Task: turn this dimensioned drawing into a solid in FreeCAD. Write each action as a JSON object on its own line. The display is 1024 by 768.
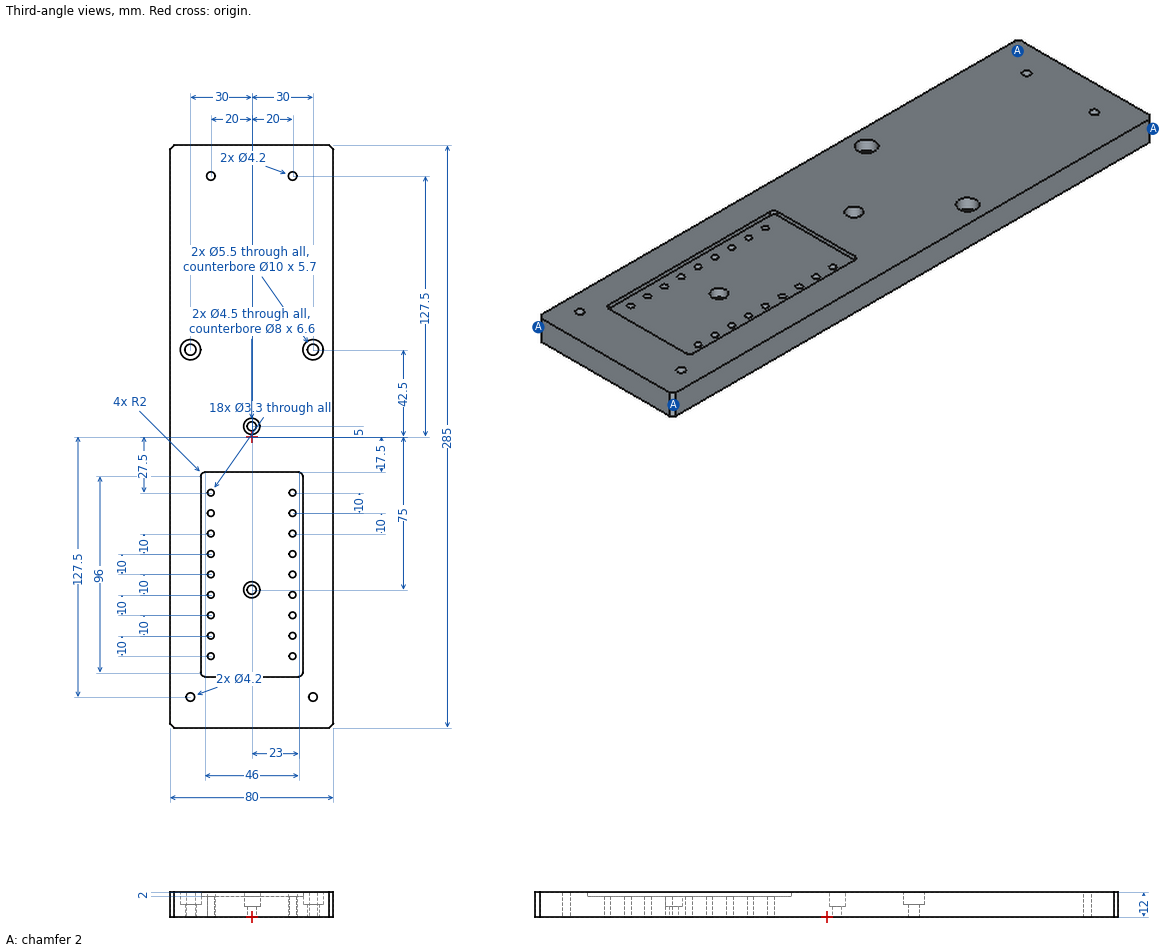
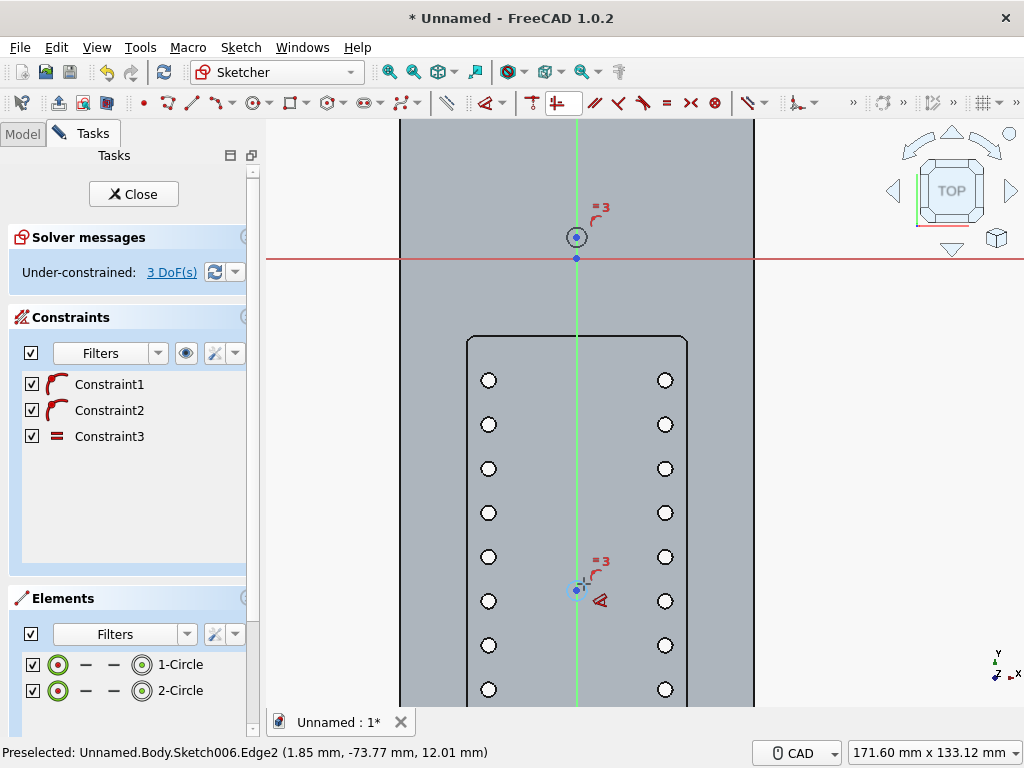
{"action": "scroll", "coordinate": [584, 230], "scroll_direction": "up", "scroll_amount": 4}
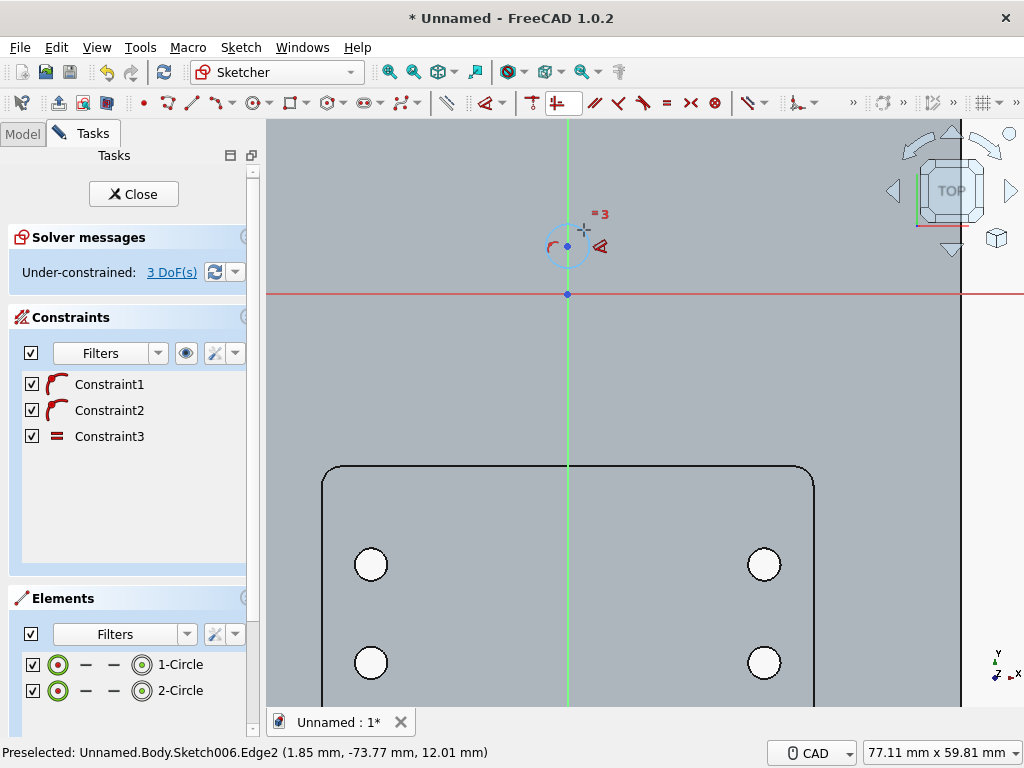
{"action": "left_click", "coordinate": [583, 231]}
{"action": "left_click", "coordinate": [606, 208]}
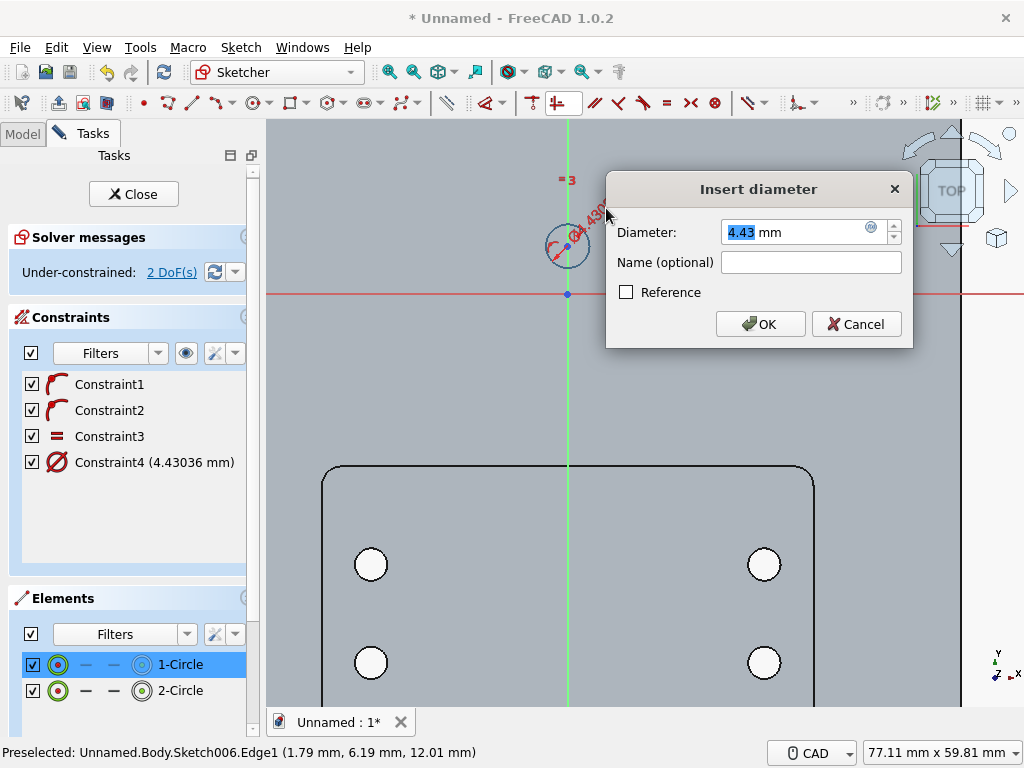
{"action": "type", "text": "4.5"}
{"action": "key", "text": "Return"}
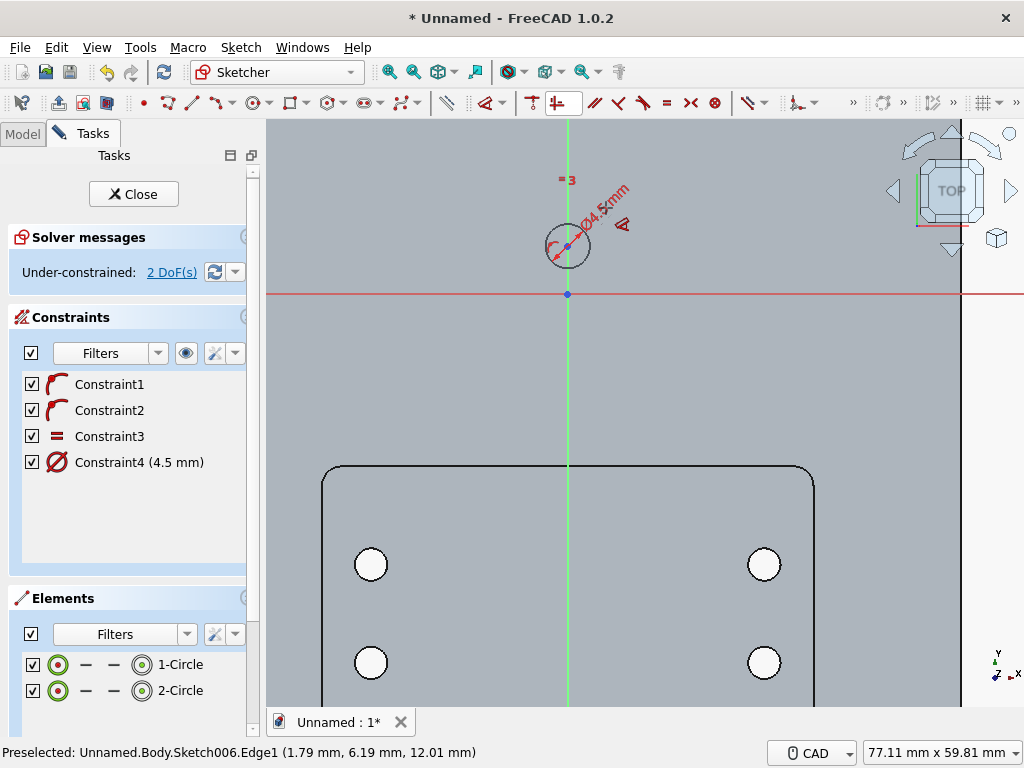
{"action": "left_click", "coordinate": [568, 246]}
{"action": "left_click", "coordinate": [602, 270]}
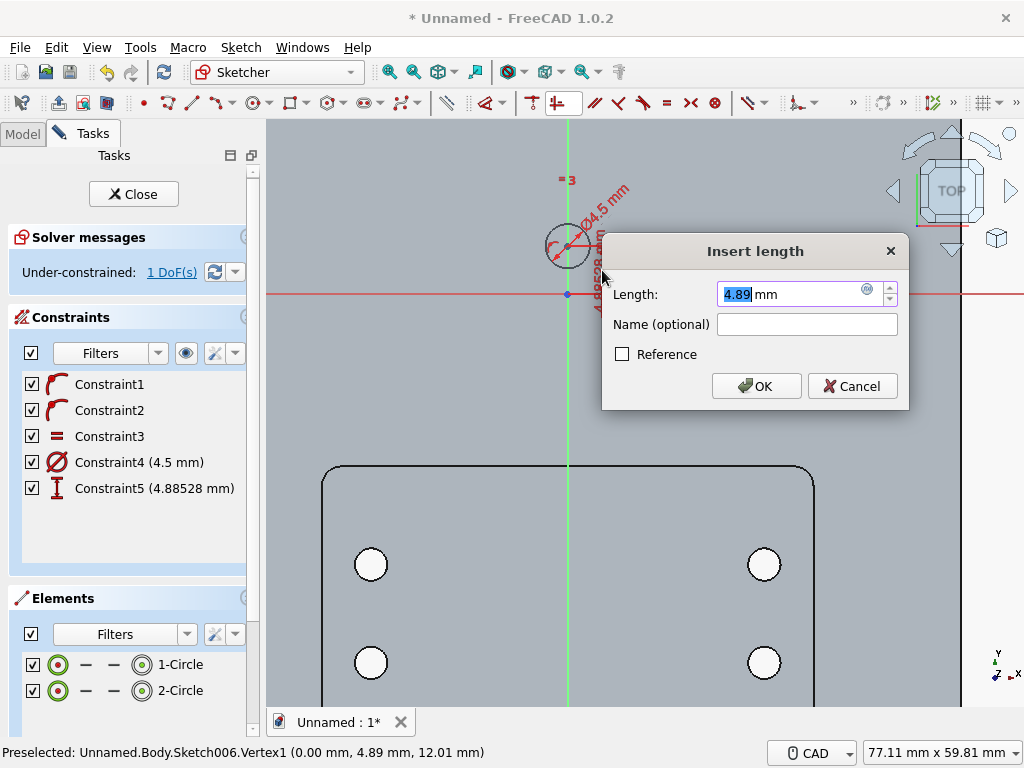
{"action": "type", "text": "5"}
{"action": "key", "text": "Return"}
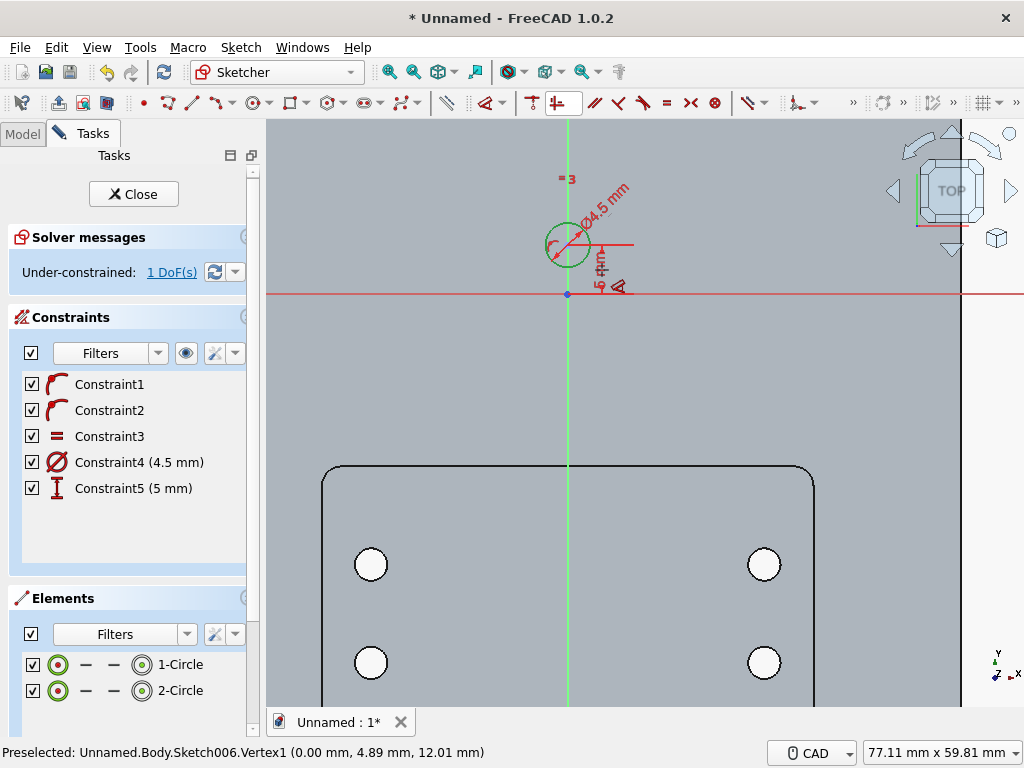
{"action": "scroll", "coordinate": [584, 229], "scroll_direction": "down", "scroll_amount": 4}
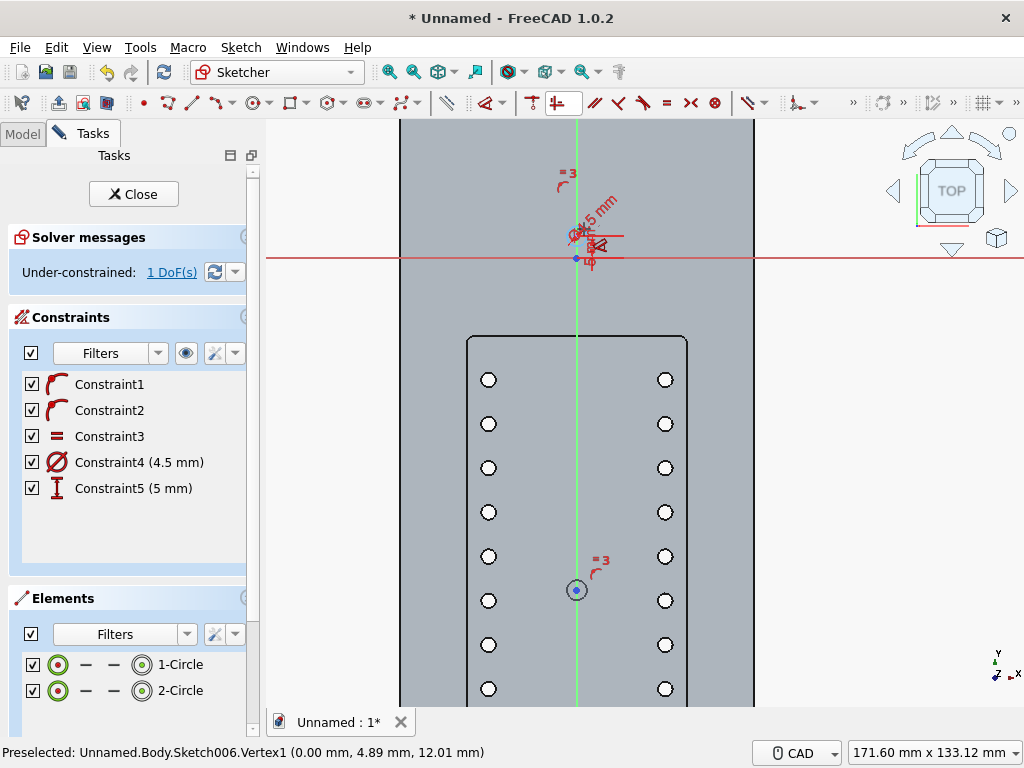
{"action": "left_click", "coordinate": [577, 590]}
{"action": "left_click", "coordinate": [611, 424]}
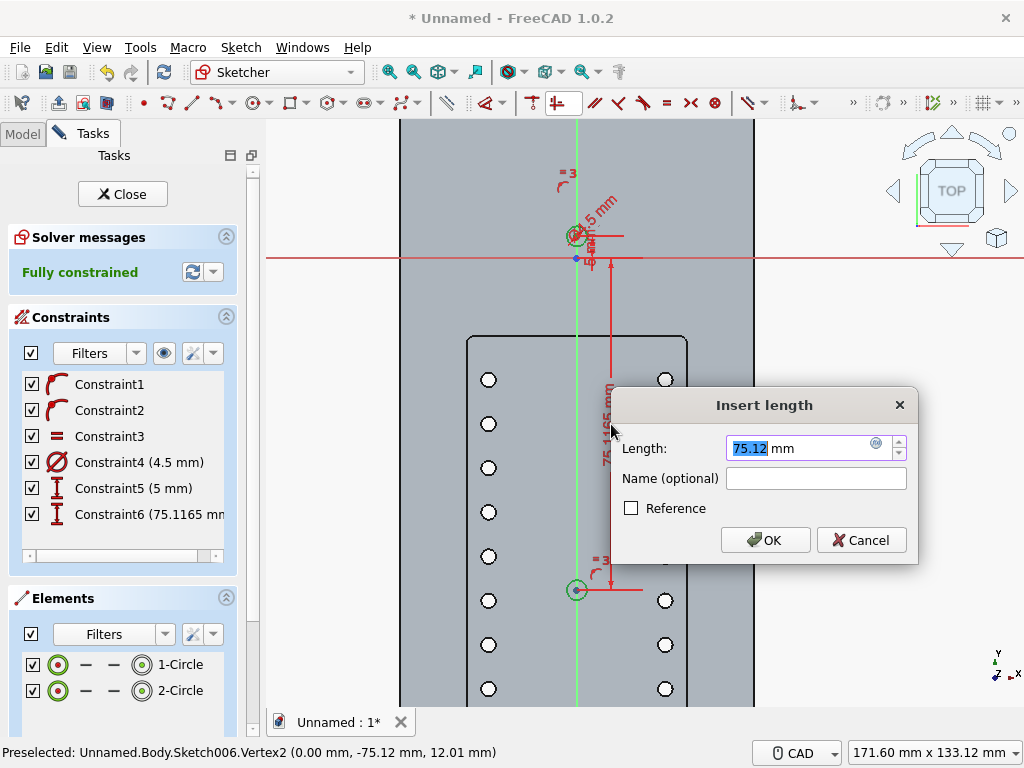
{"action": "type", "text": "75"}
{"action": "key", "text": "Return"}
{"action": "key", "text": "Escape"}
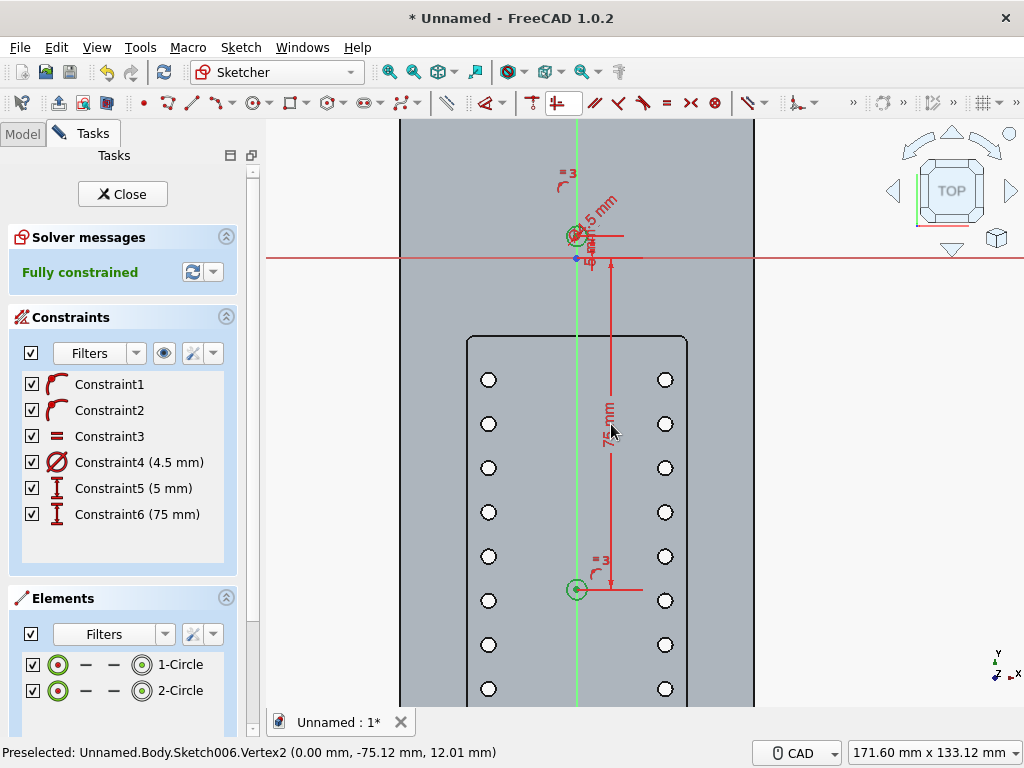
{"action": "left_click", "coordinate": [123, 194]}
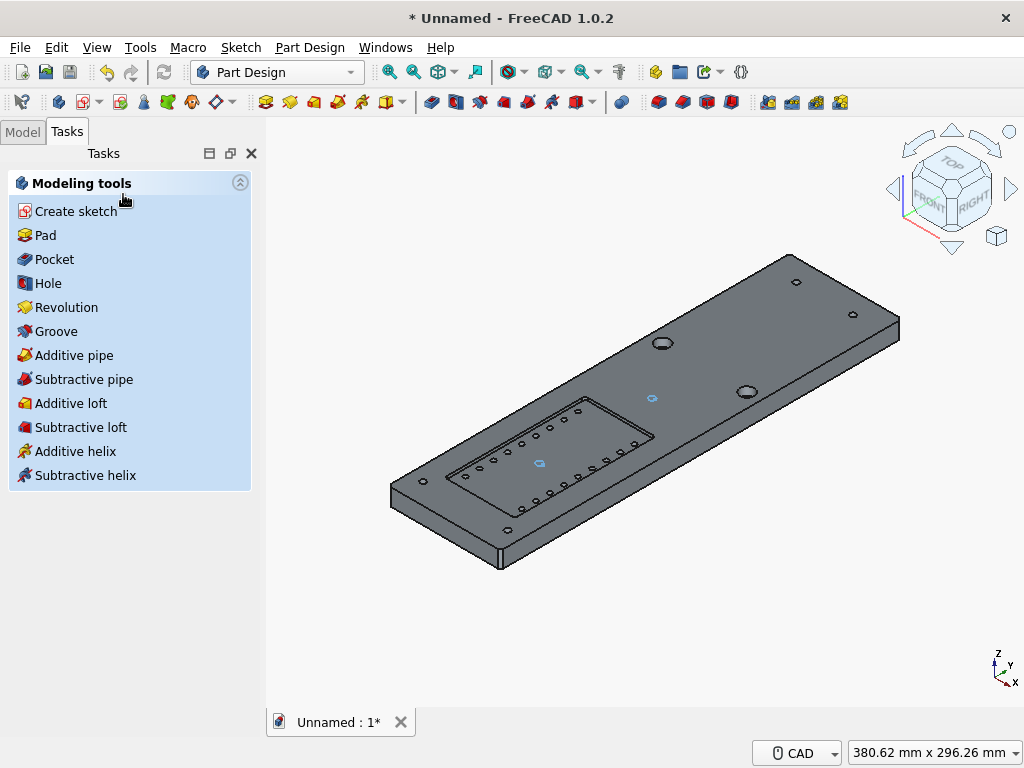
{"action": "left_click", "coordinate": [456, 102]}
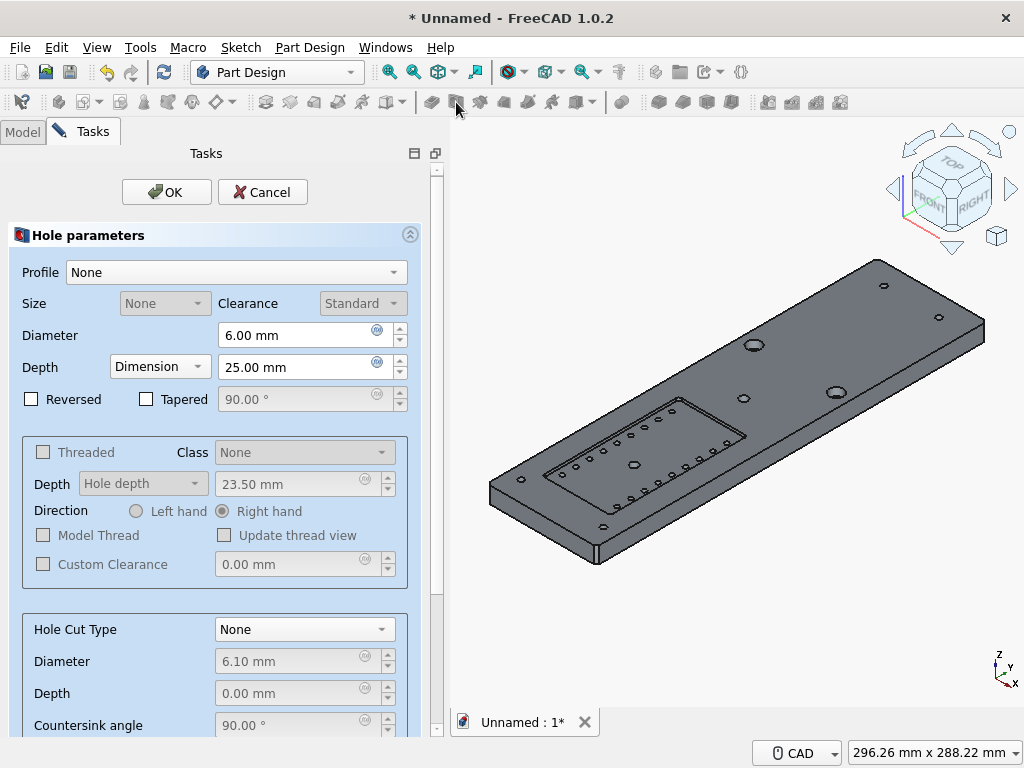
{"action": "triple_click", "coordinate": [305, 335]}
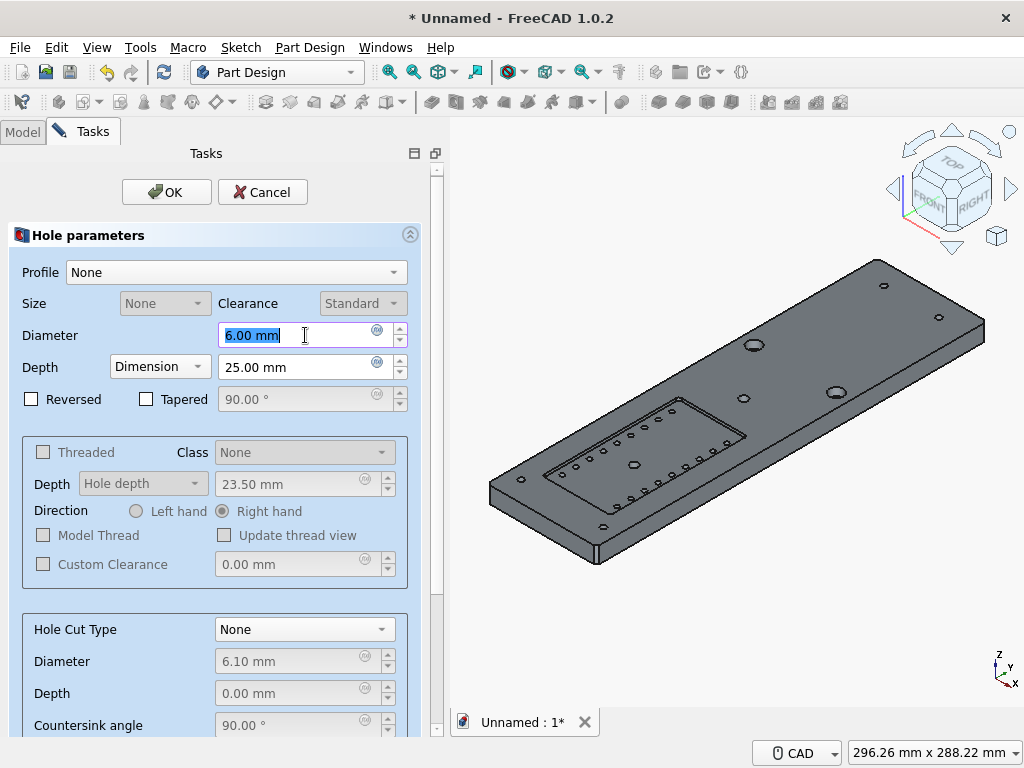
{"action": "type", "text": "4.5"}
{"action": "key", "text": "Tab"}